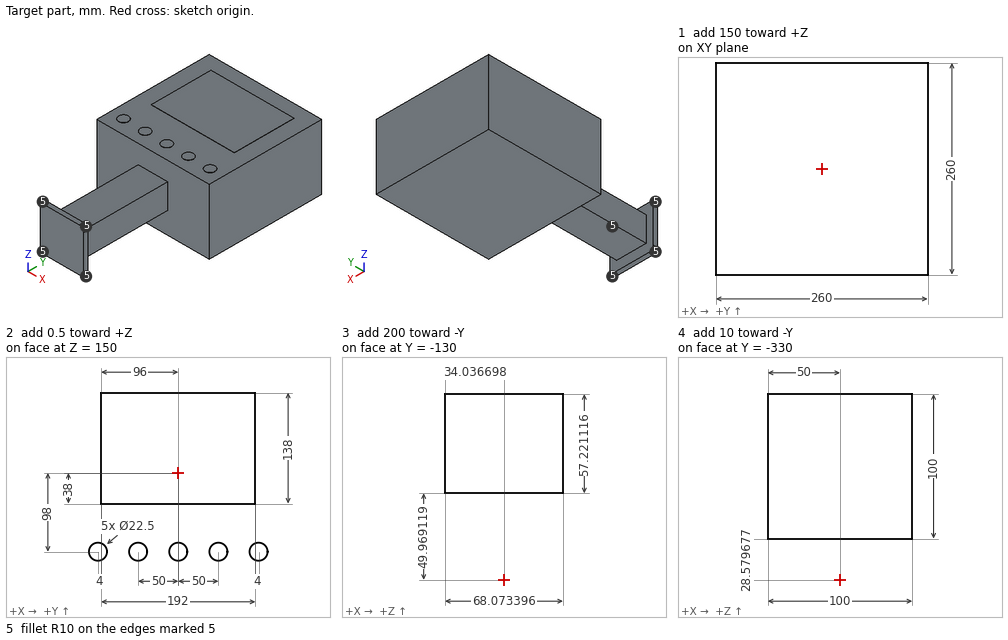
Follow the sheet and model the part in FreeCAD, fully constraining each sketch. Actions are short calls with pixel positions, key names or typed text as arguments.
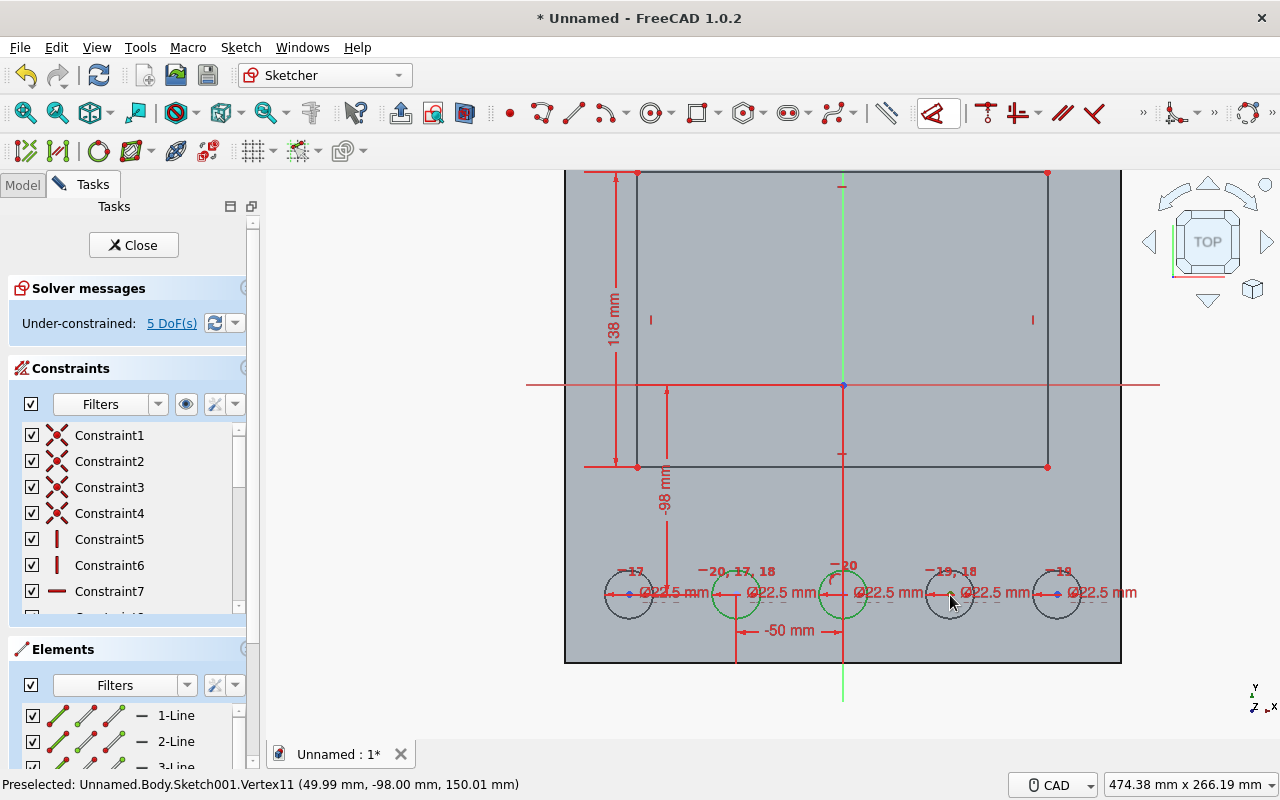
click(954, 114)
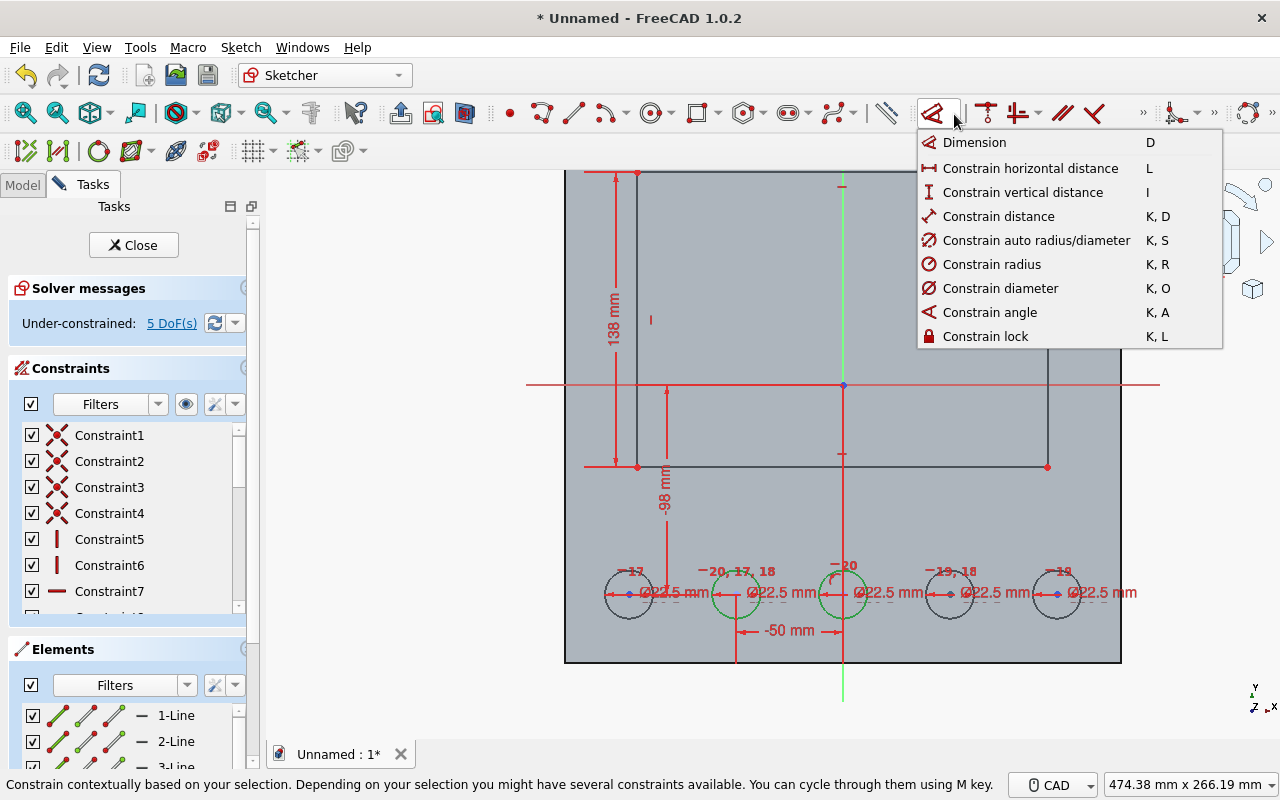
click(1070, 168)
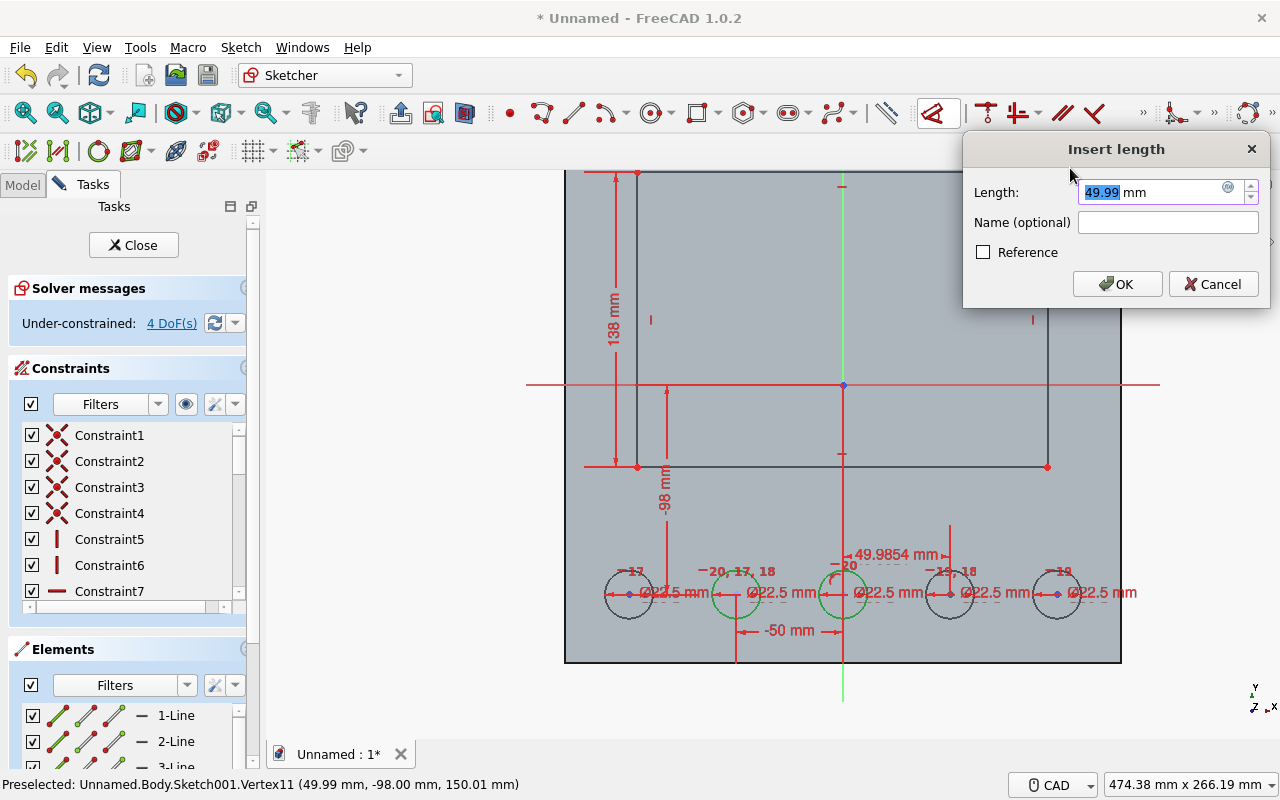
text(50)
key(Return)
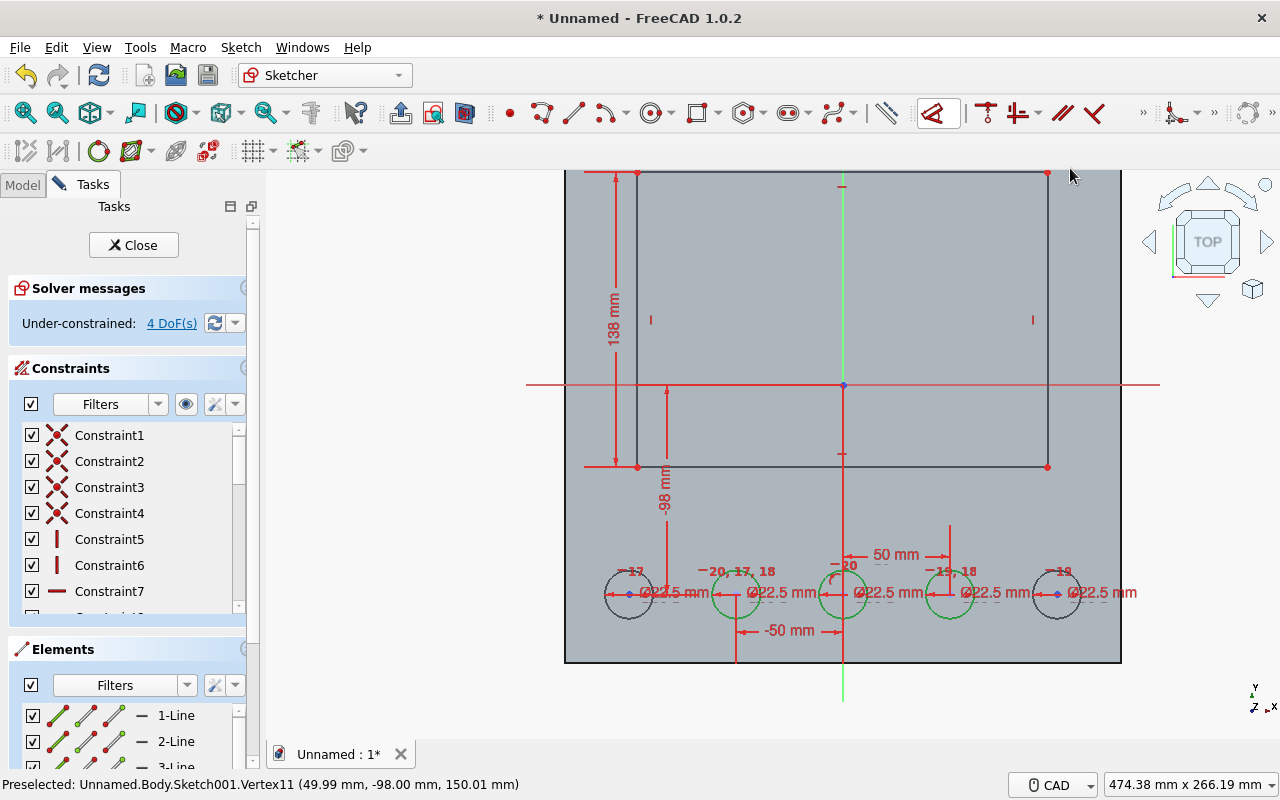
scroll(637, 467, up, 8)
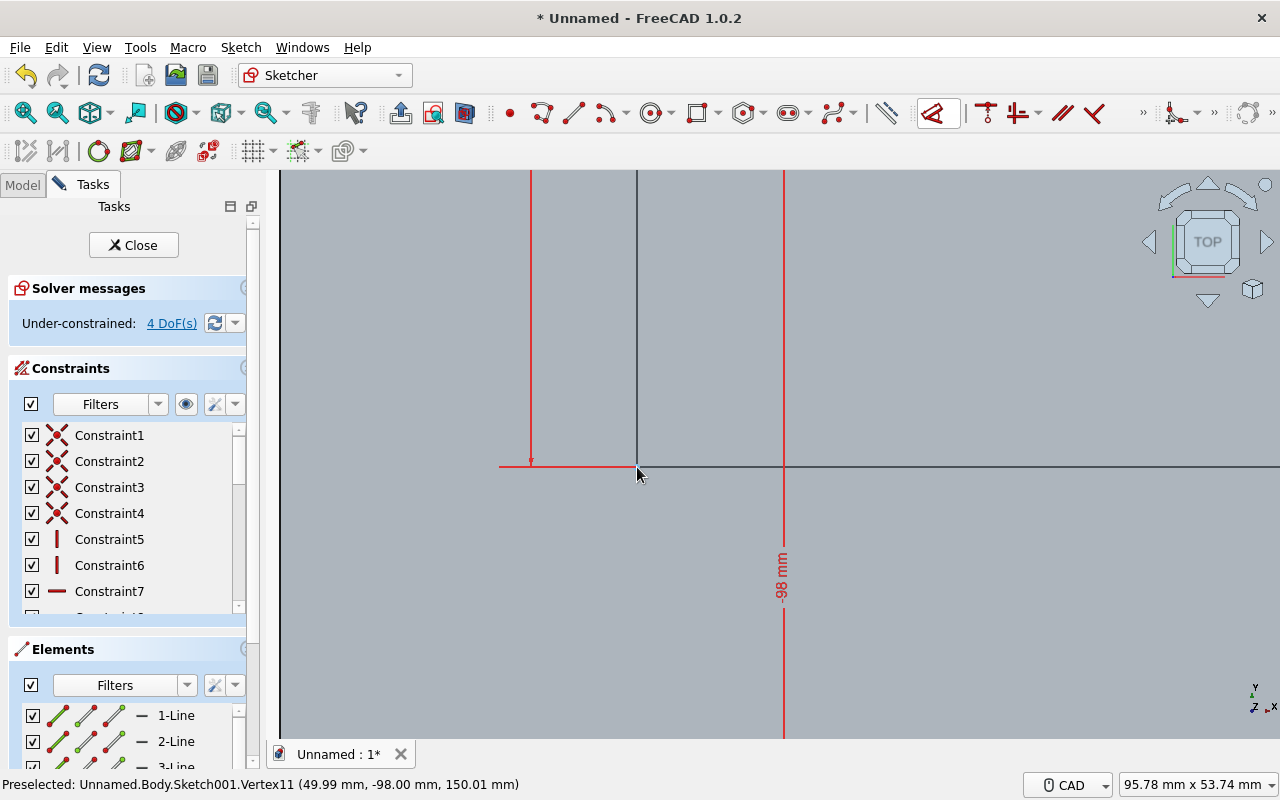
click(637, 467)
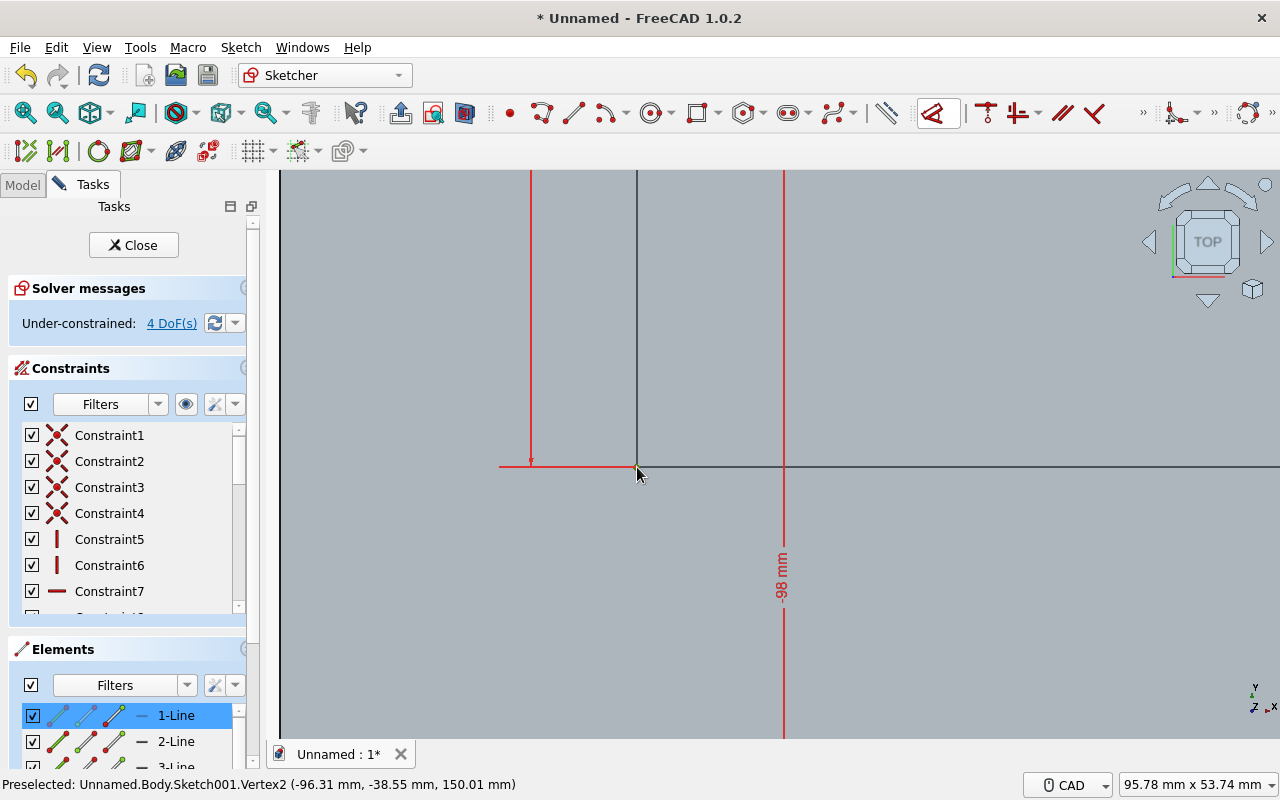
scroll(516, 523, down, 9)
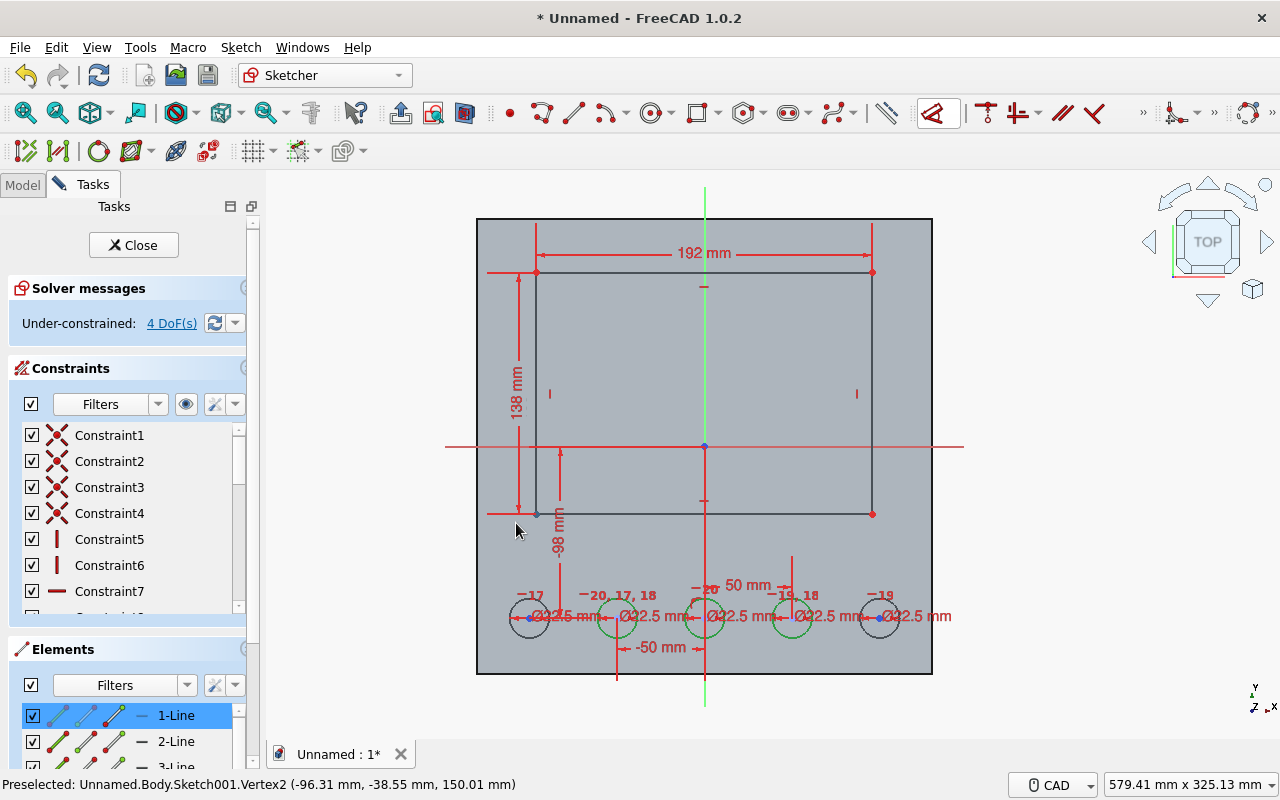
scroll(529, 618, up, 9)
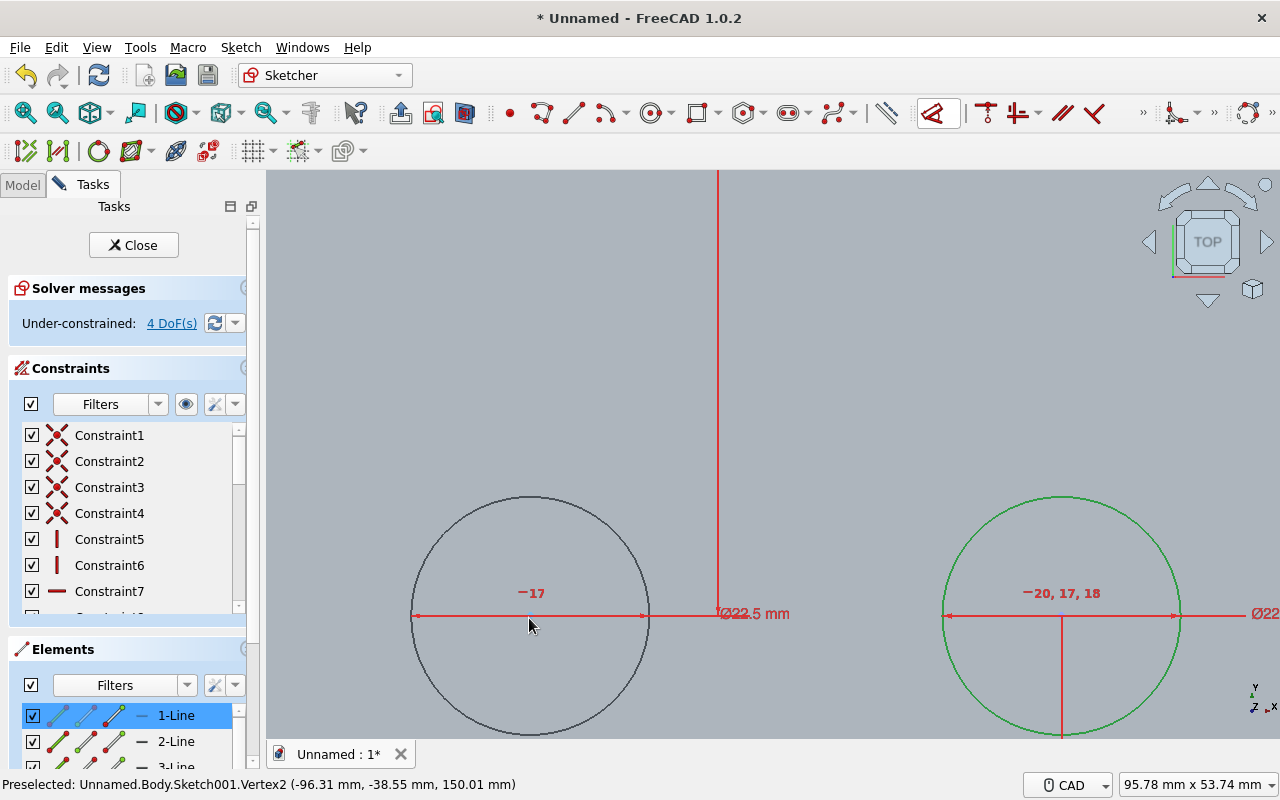
click(530, 616)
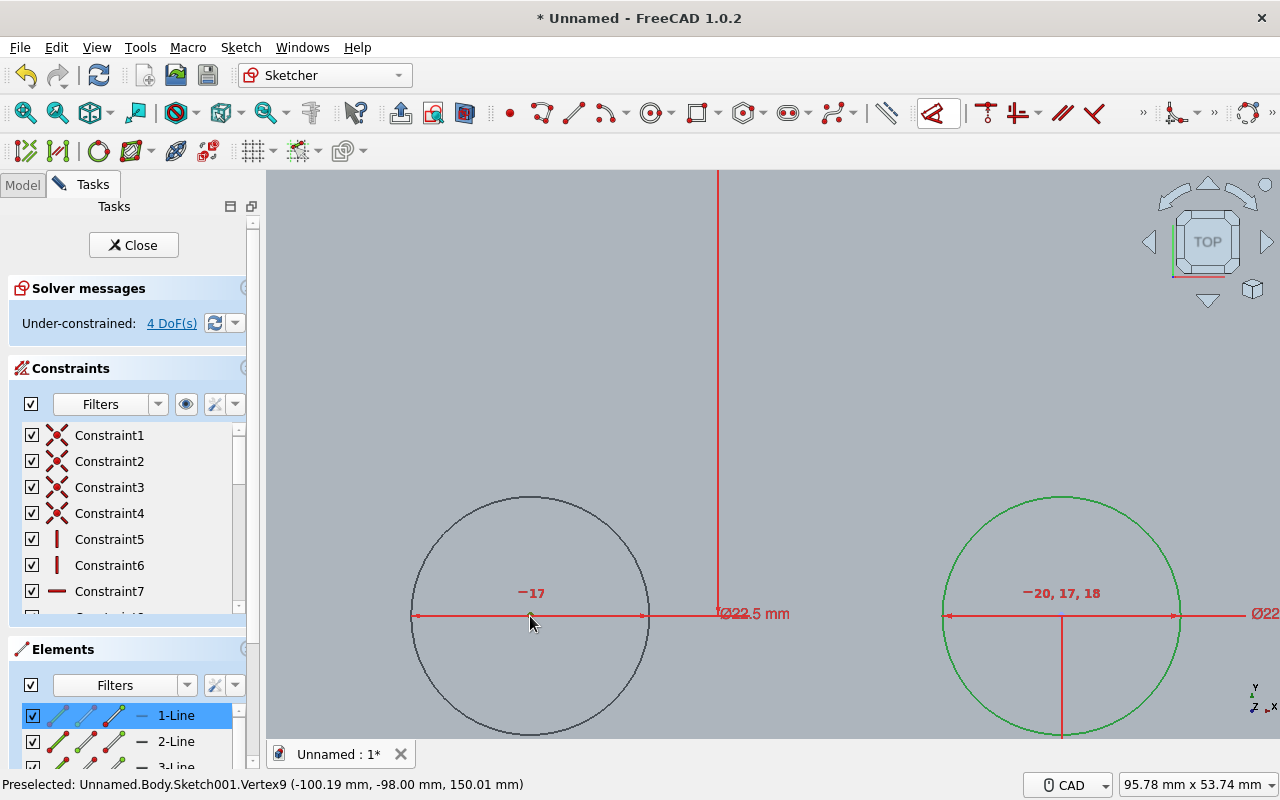
key(l)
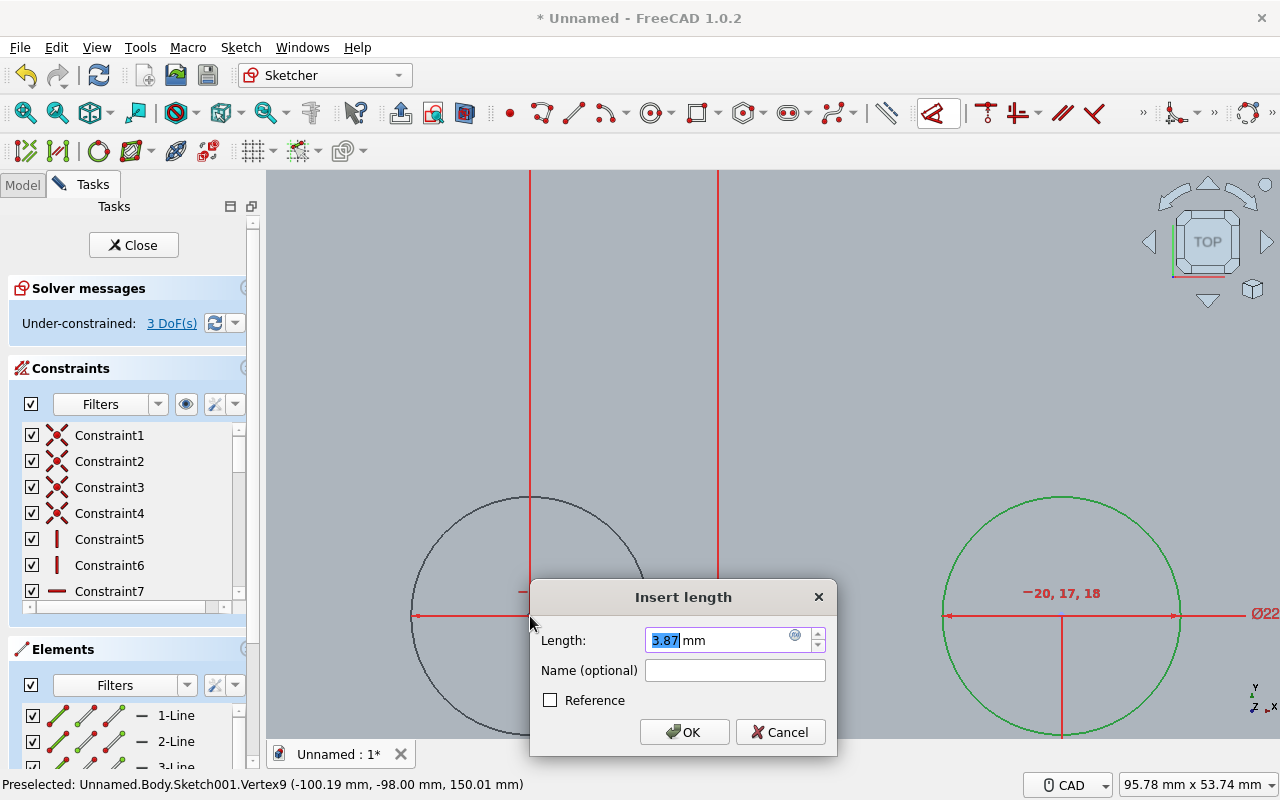
text(4)
key(Return)